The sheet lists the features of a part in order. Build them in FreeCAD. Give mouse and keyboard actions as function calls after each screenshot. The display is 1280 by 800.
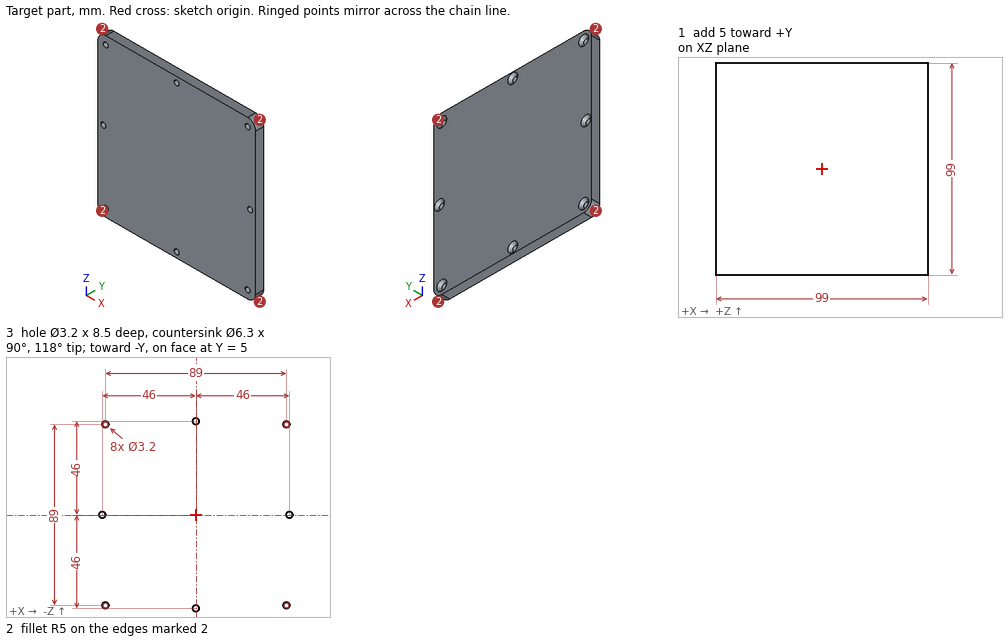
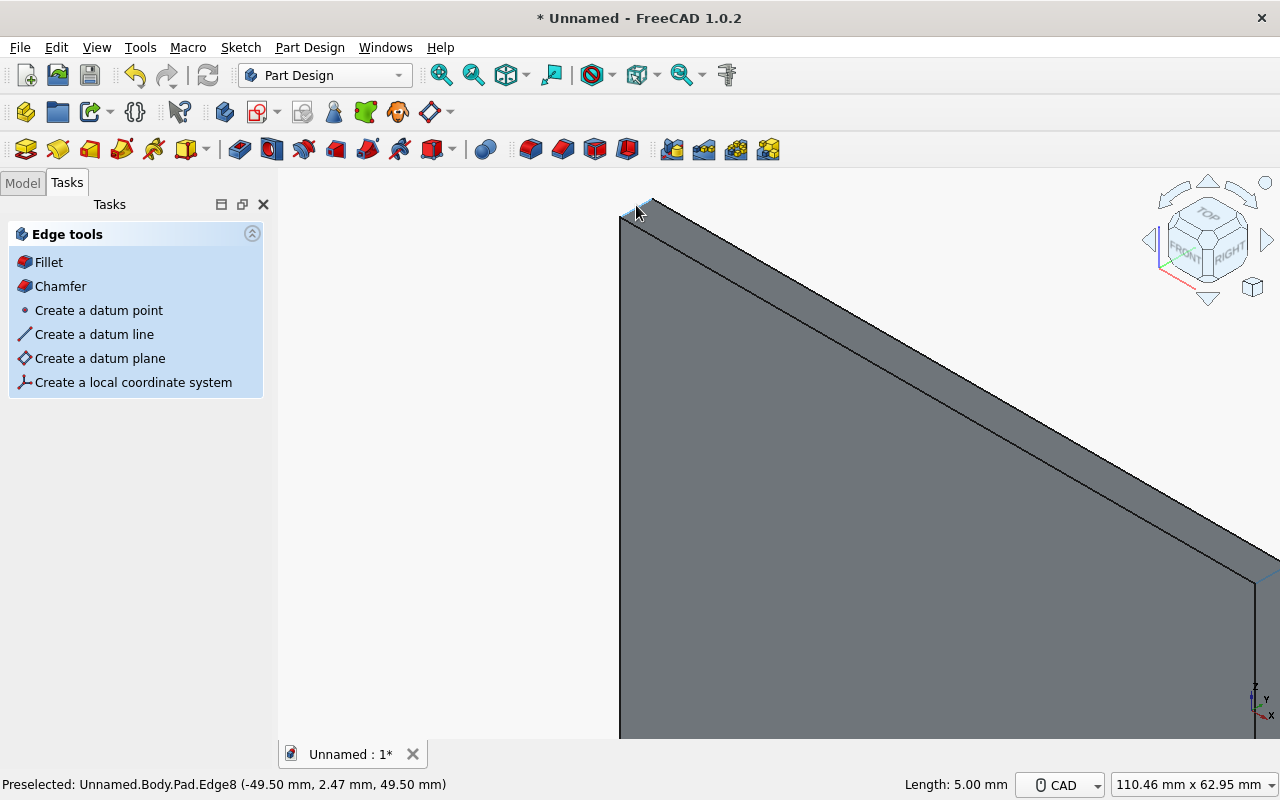
key(v)
key(f)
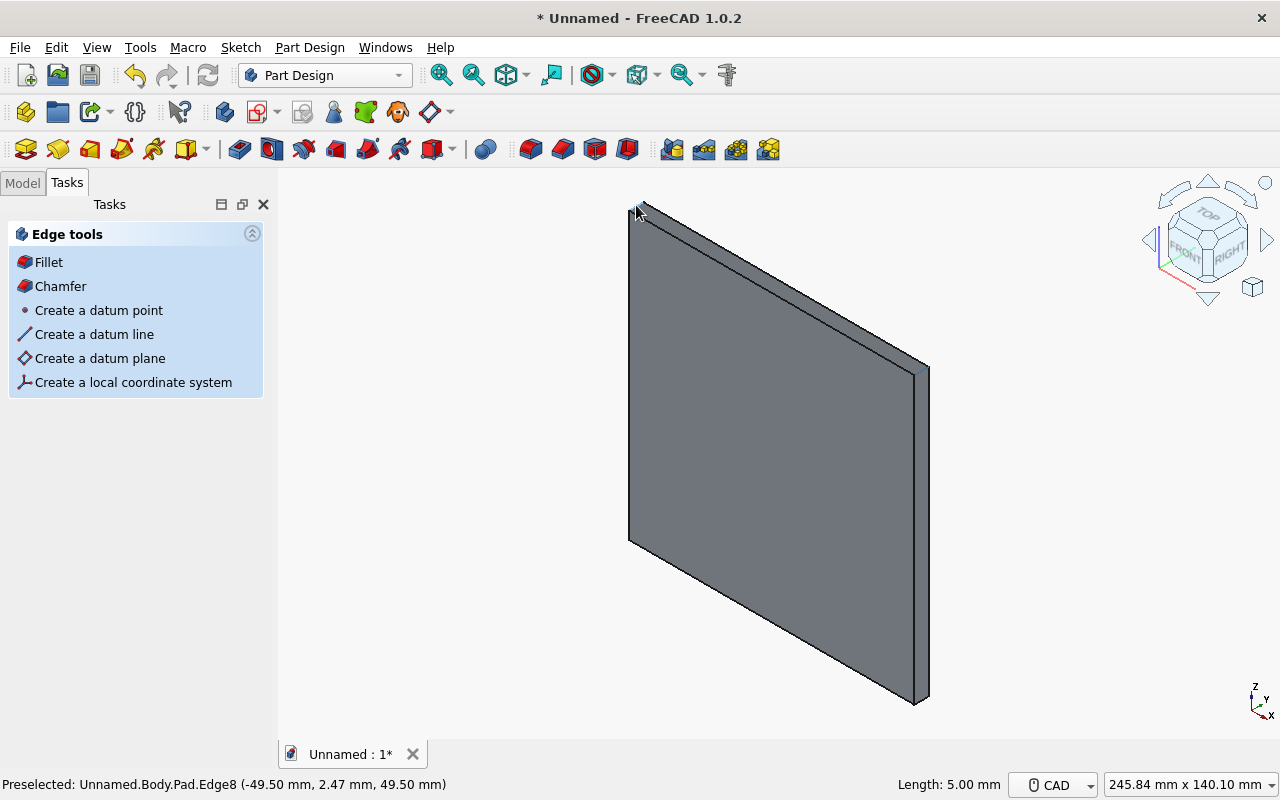
key(2)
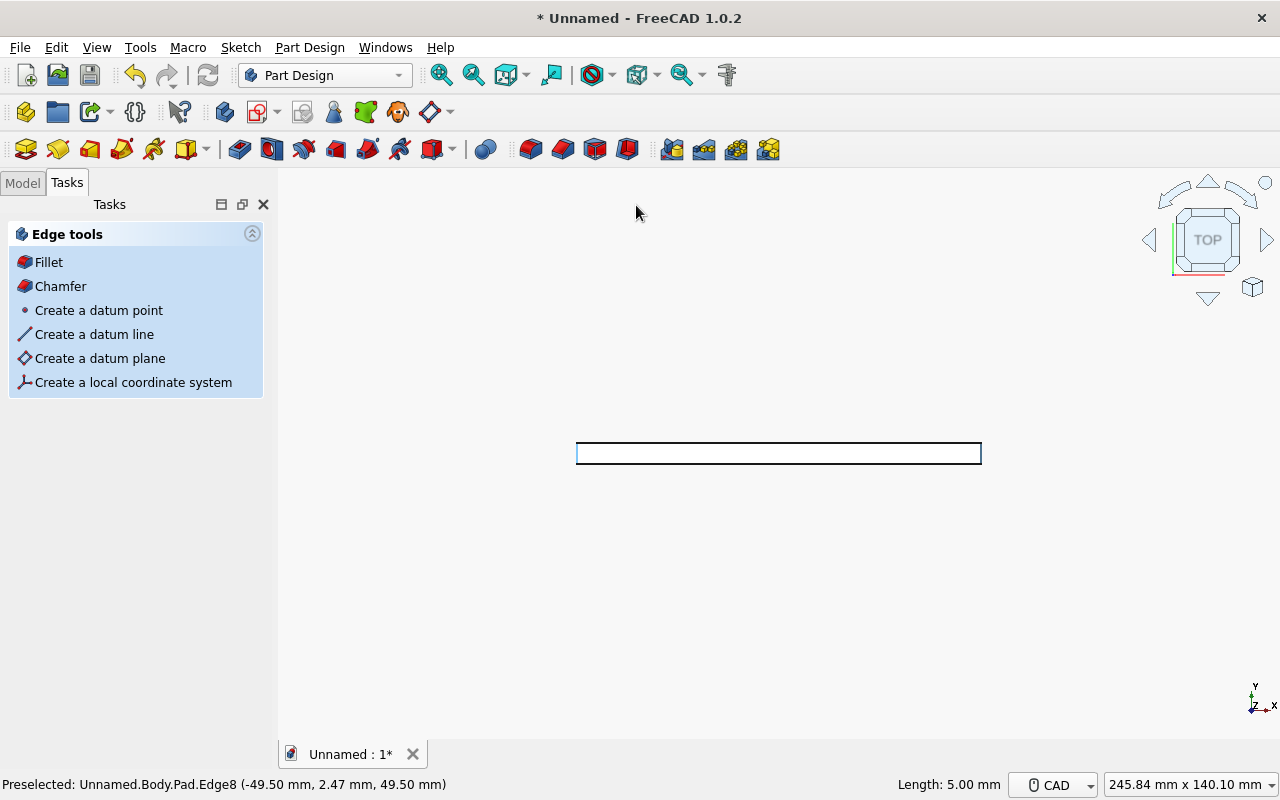
key(v)
key(f)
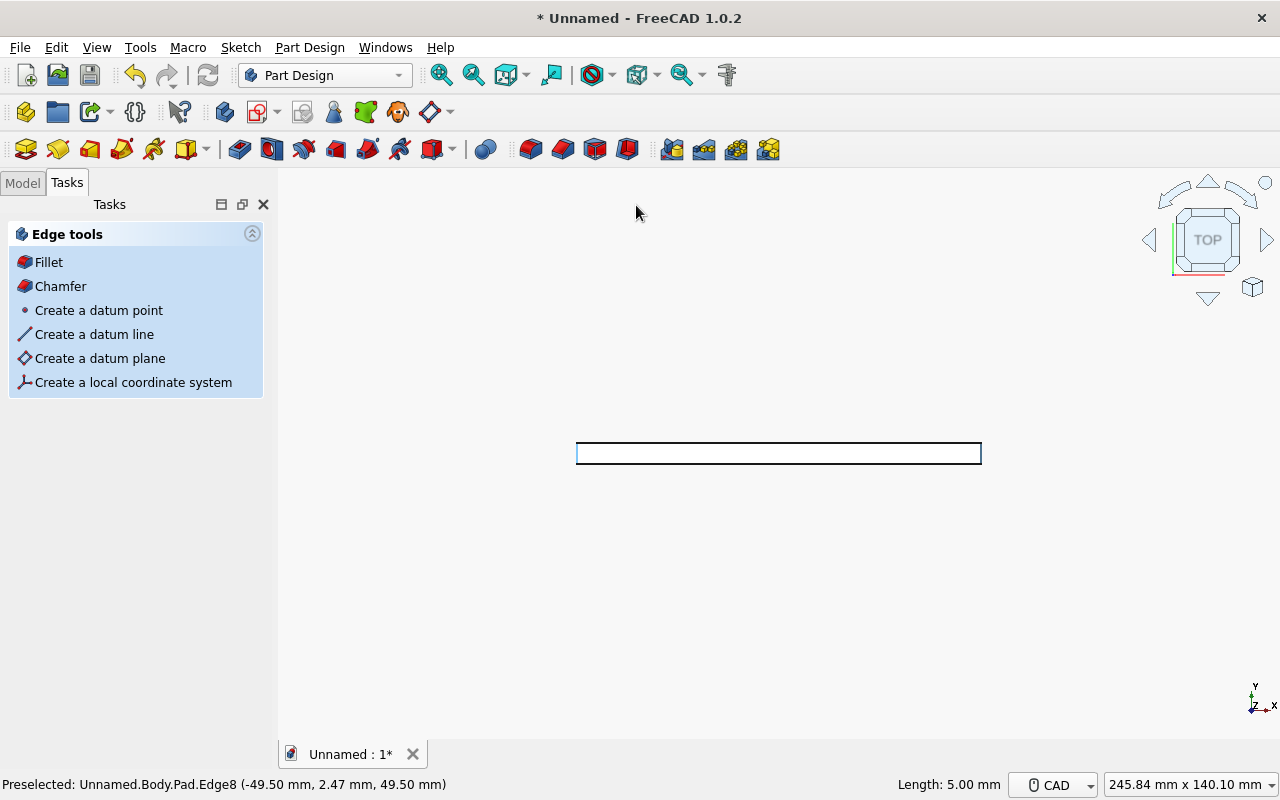
click(577, 452, ctrl)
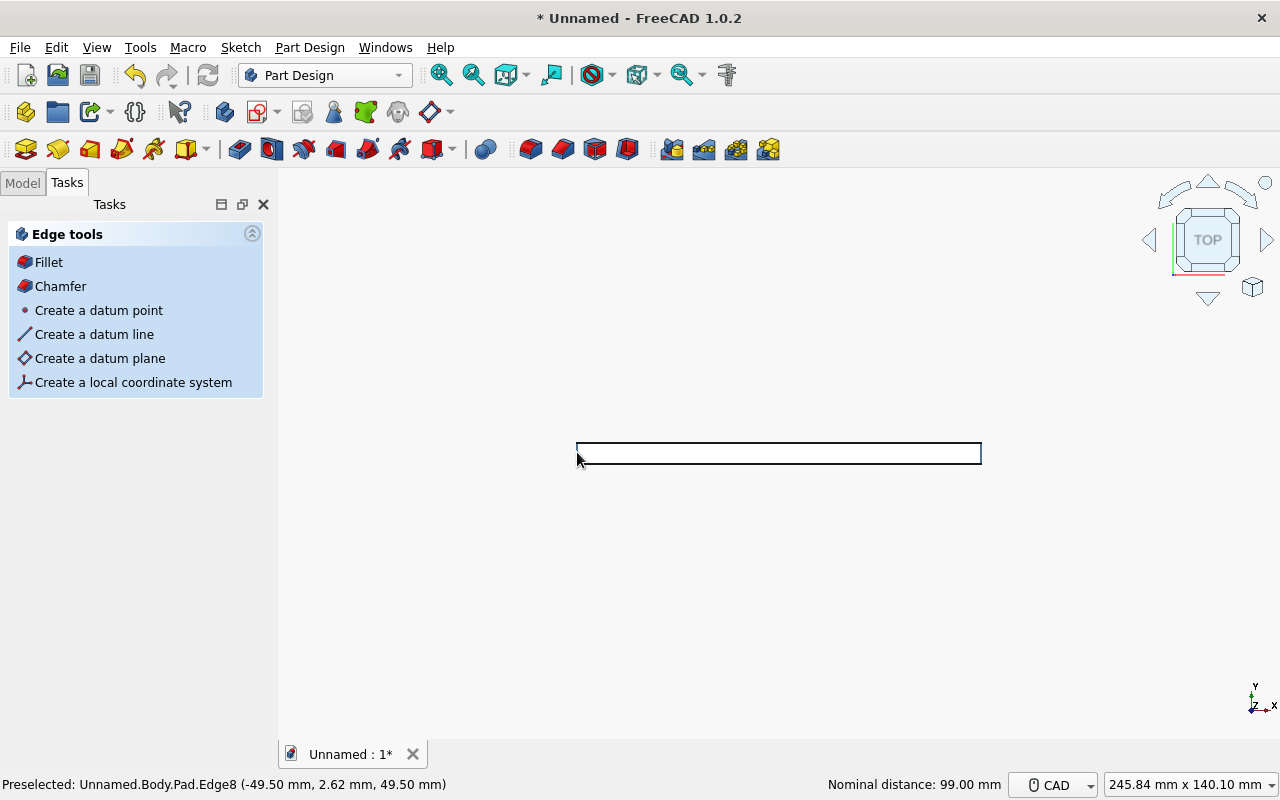
scroll(577, 452, up, 4)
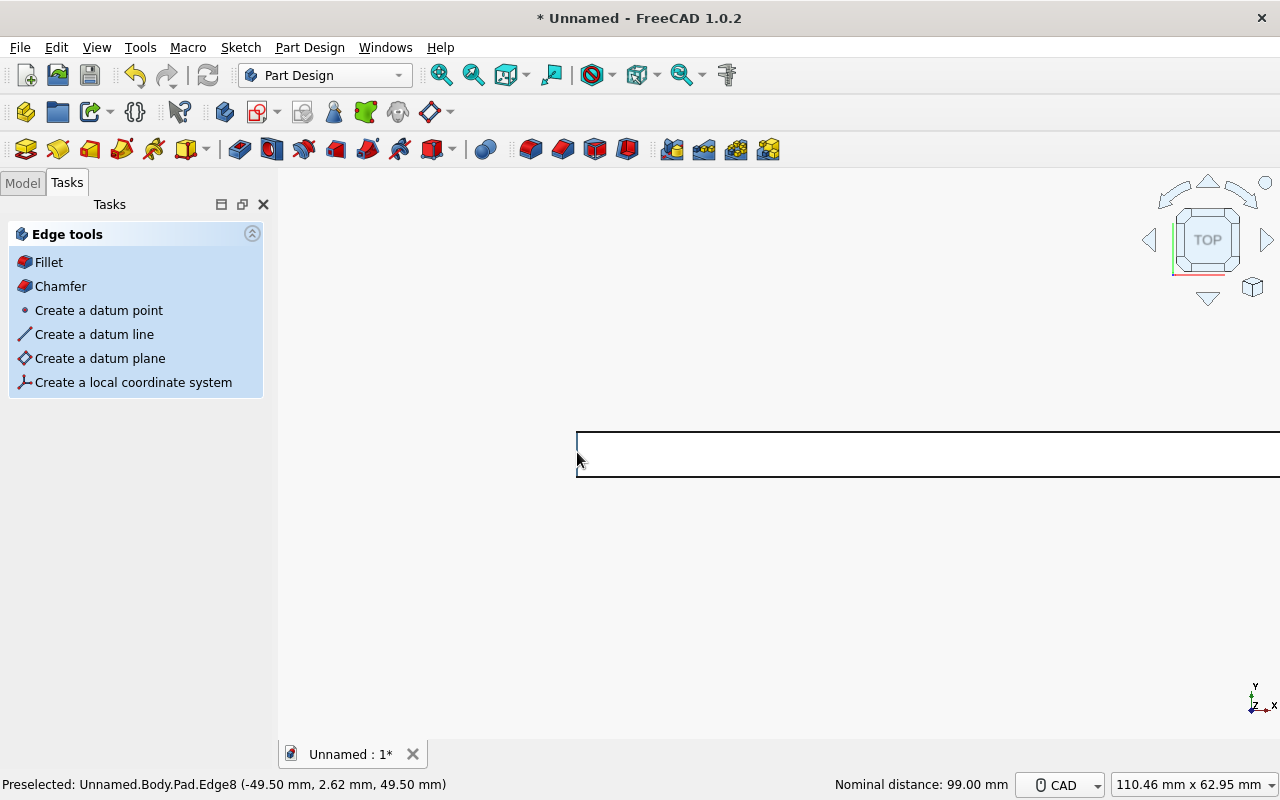
key(v)
key(f)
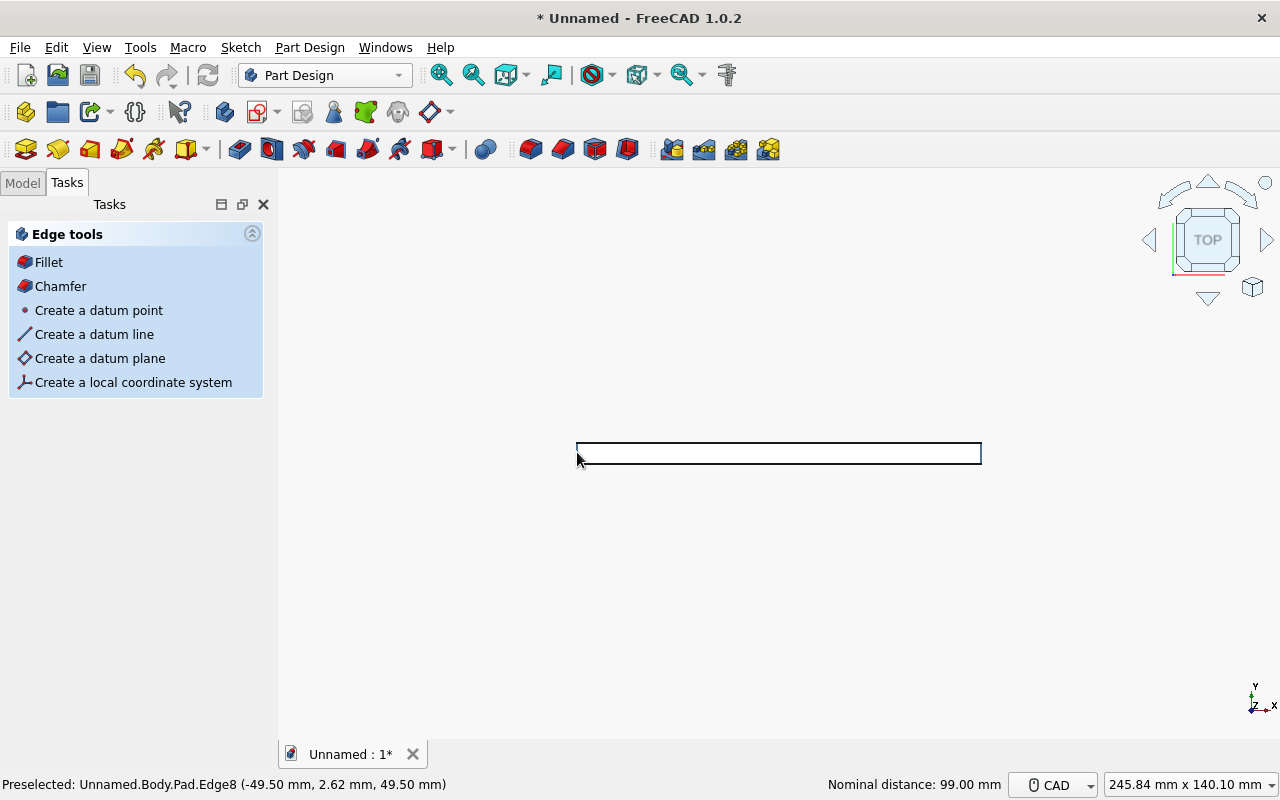
key(1)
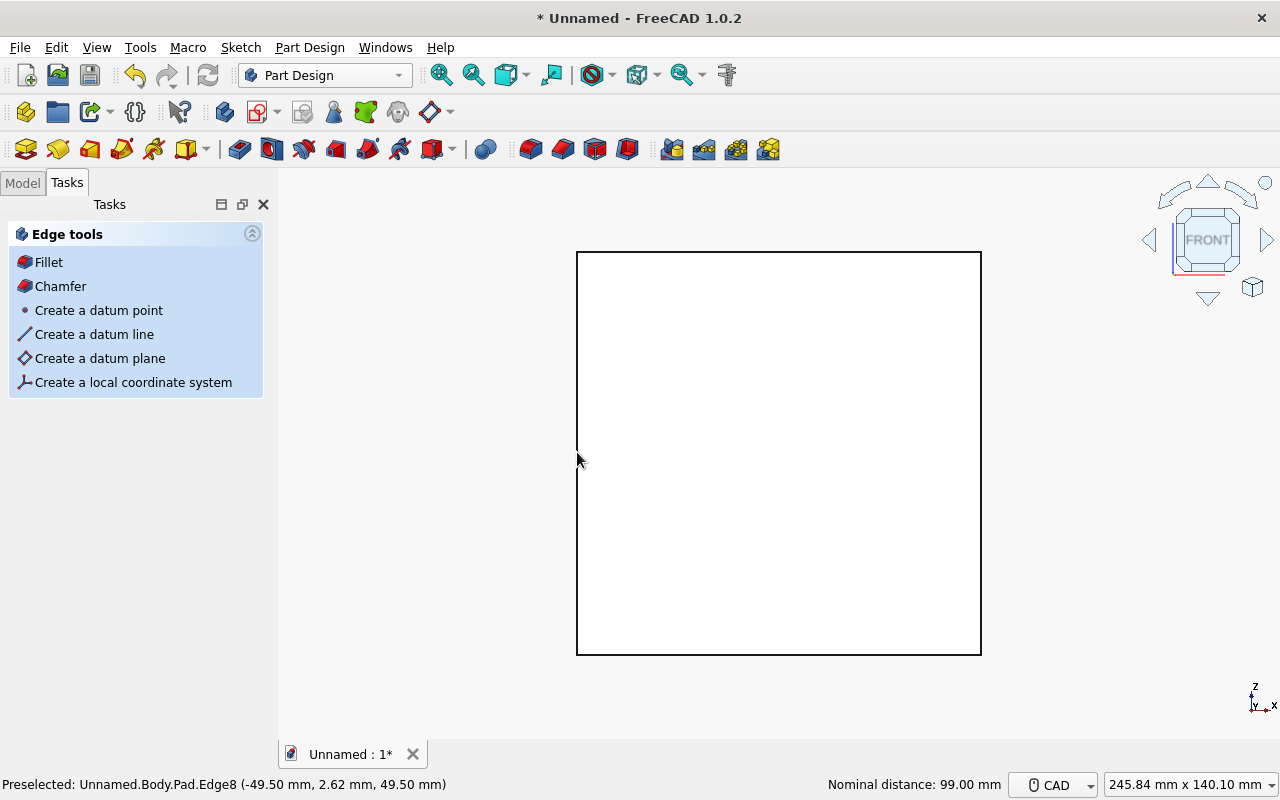
scroll(577, 654, up, 4)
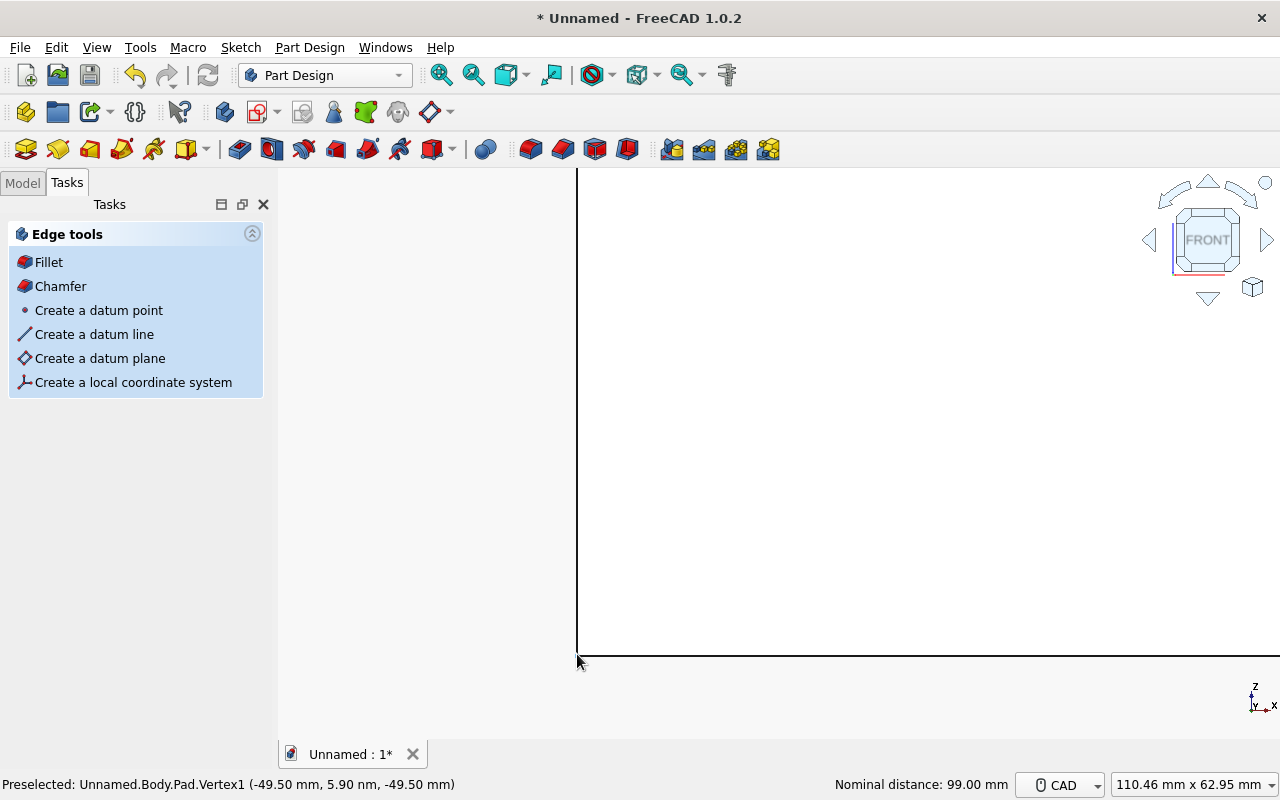
key(v)
key(f)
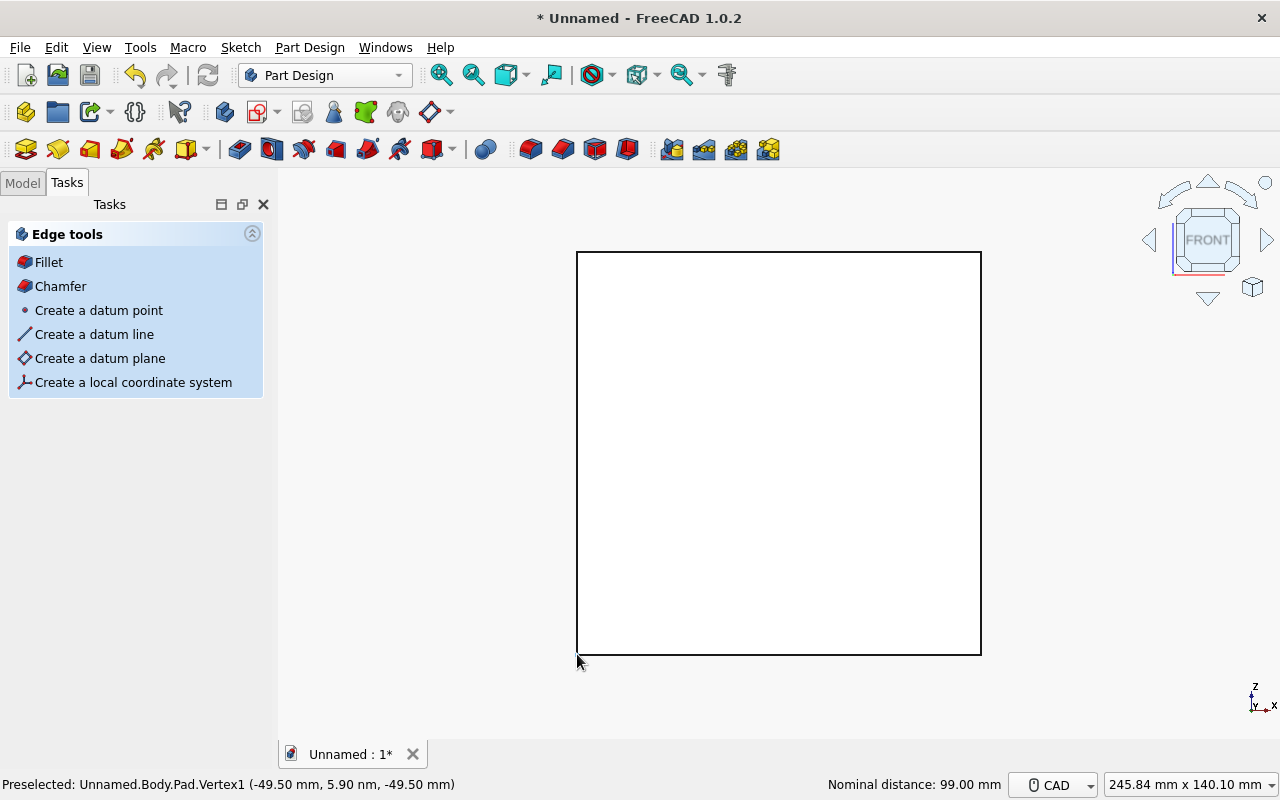
key(3)